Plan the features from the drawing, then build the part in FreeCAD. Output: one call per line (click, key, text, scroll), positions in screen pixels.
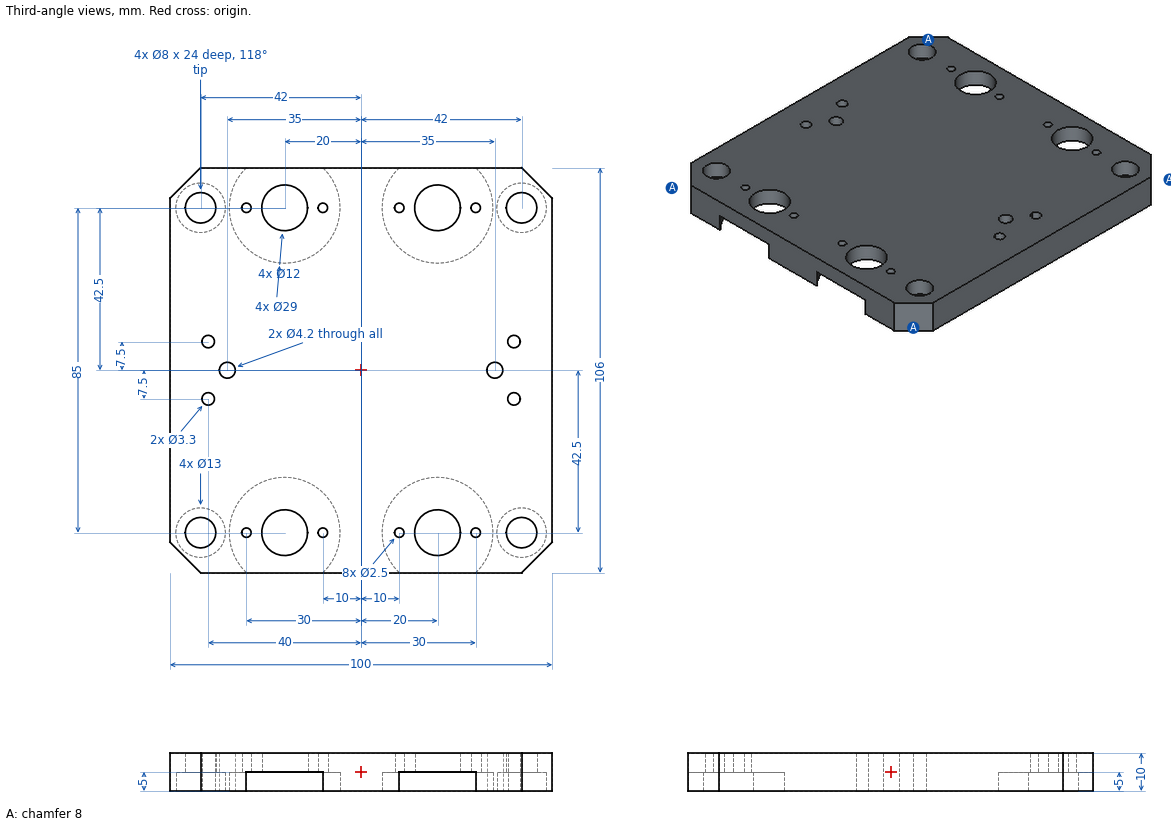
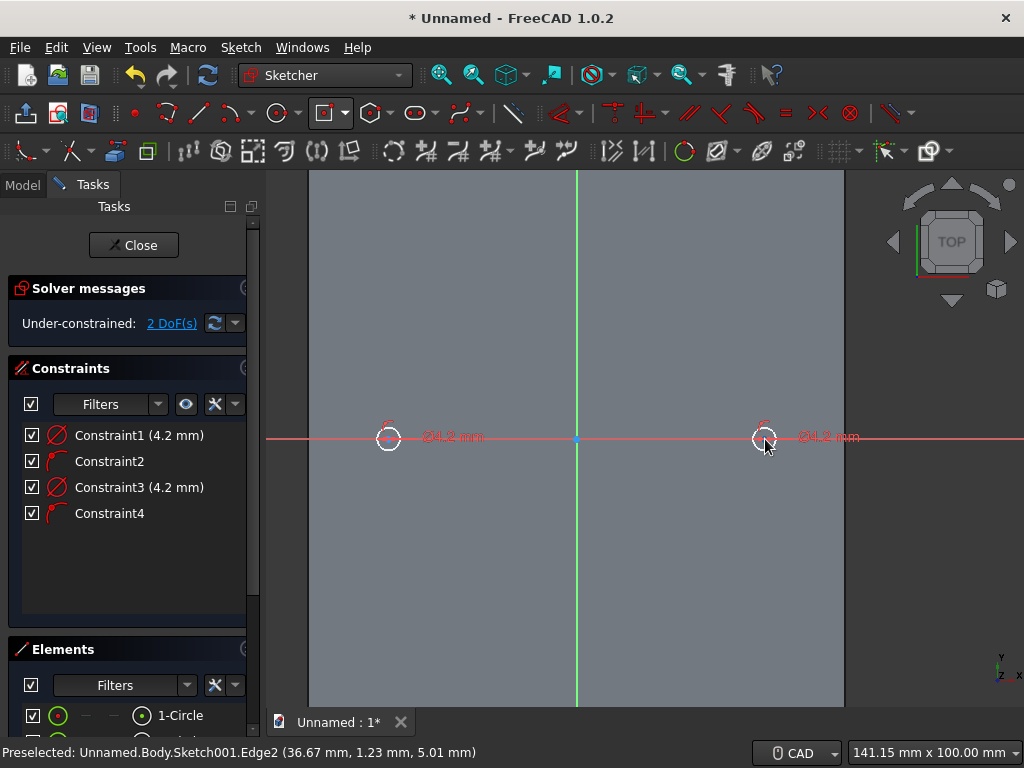
click(389, 439)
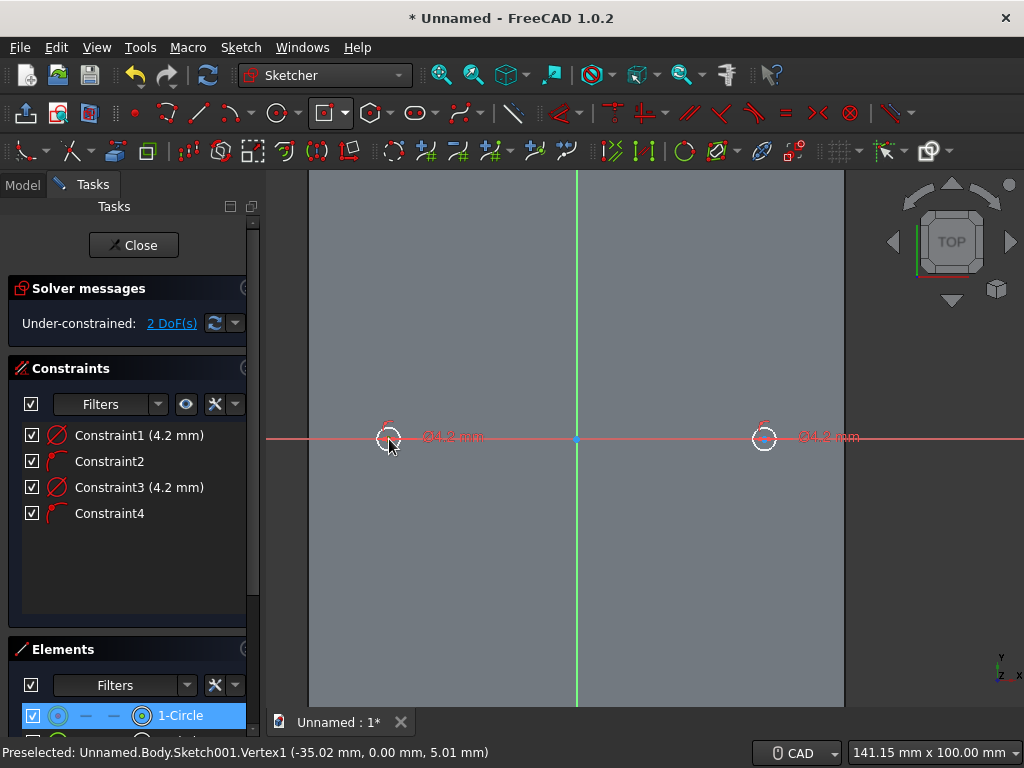
click(582, 114)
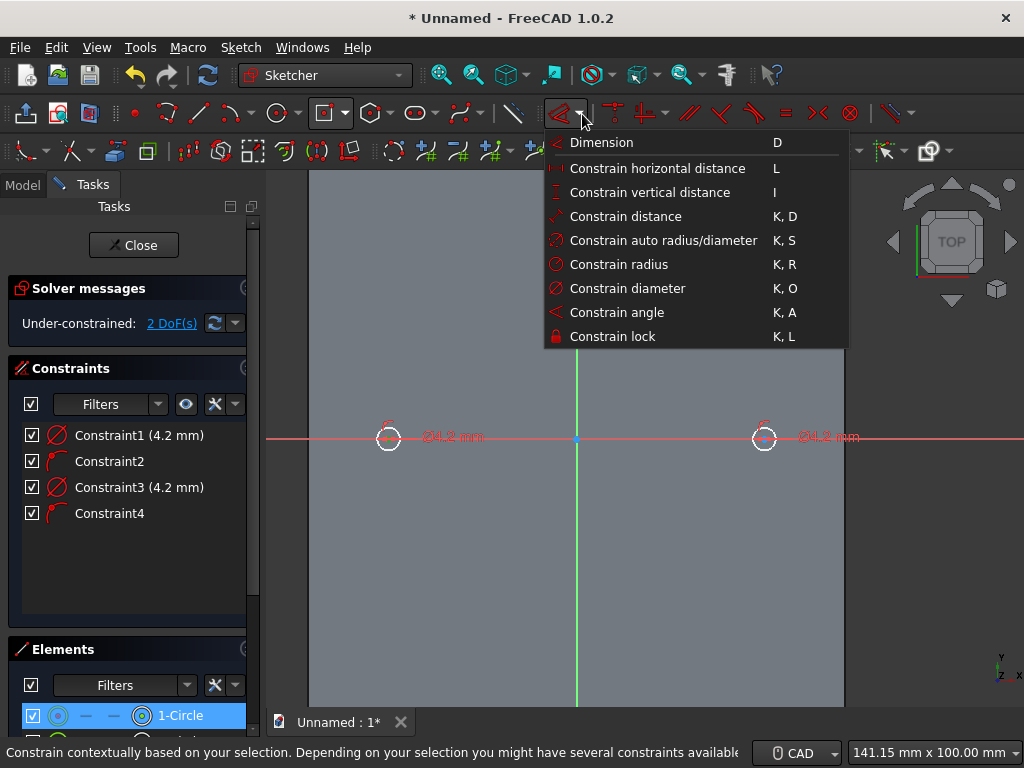
click(697, 168)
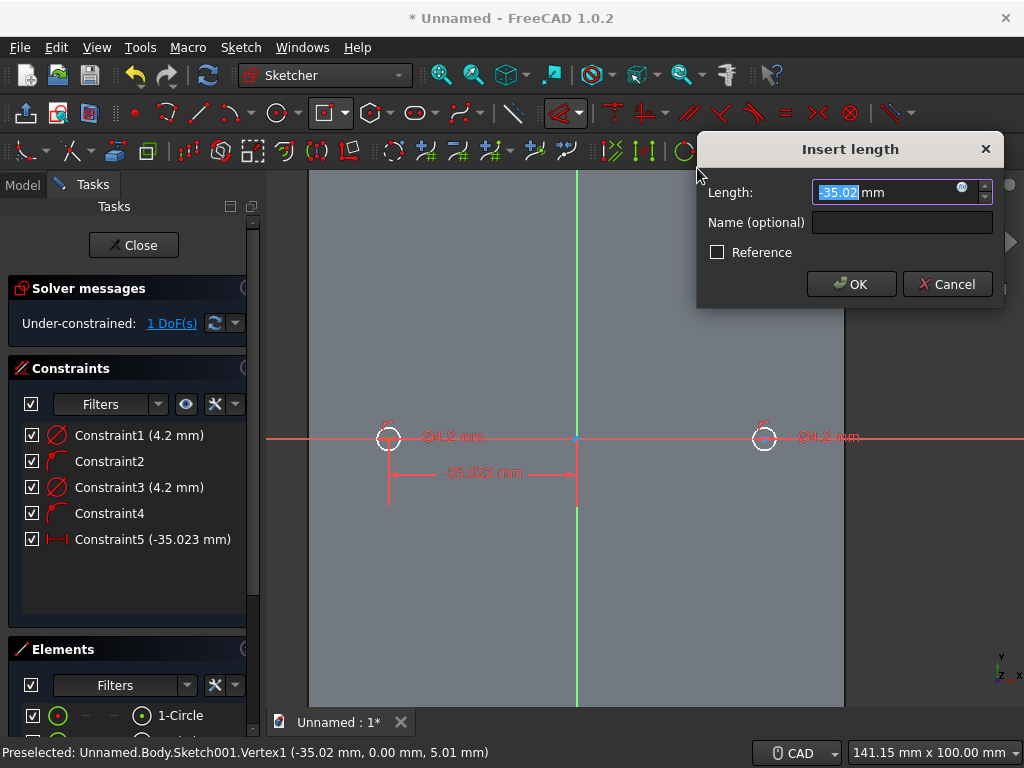
text(-35)
key(Return)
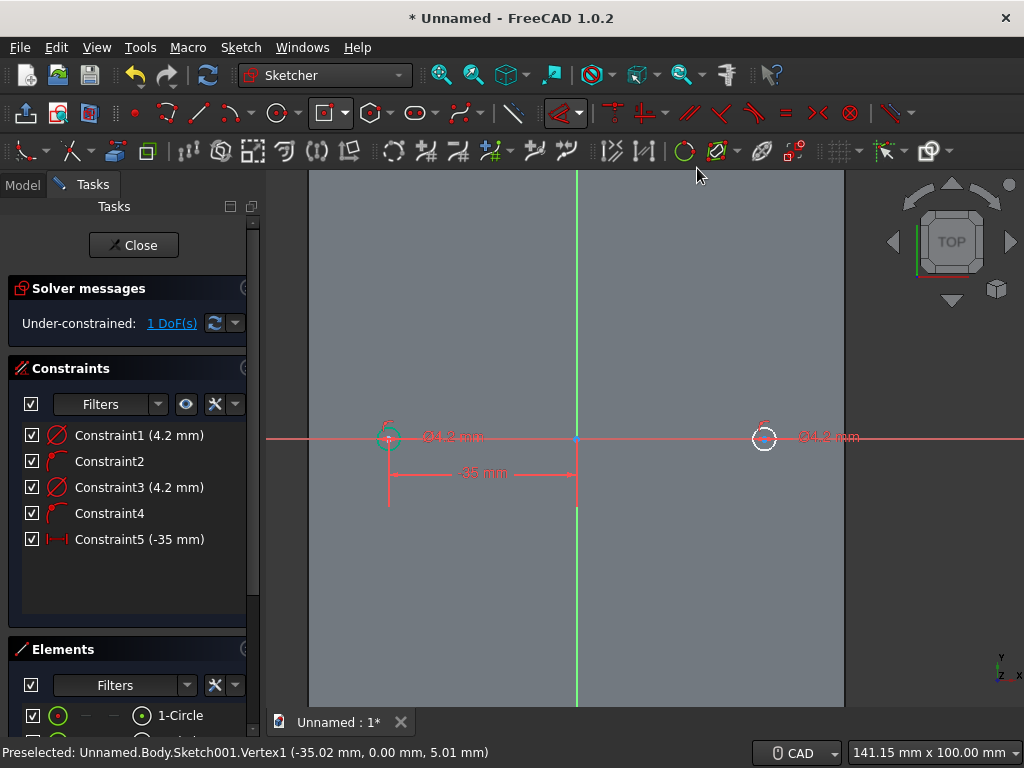
click(764, 439)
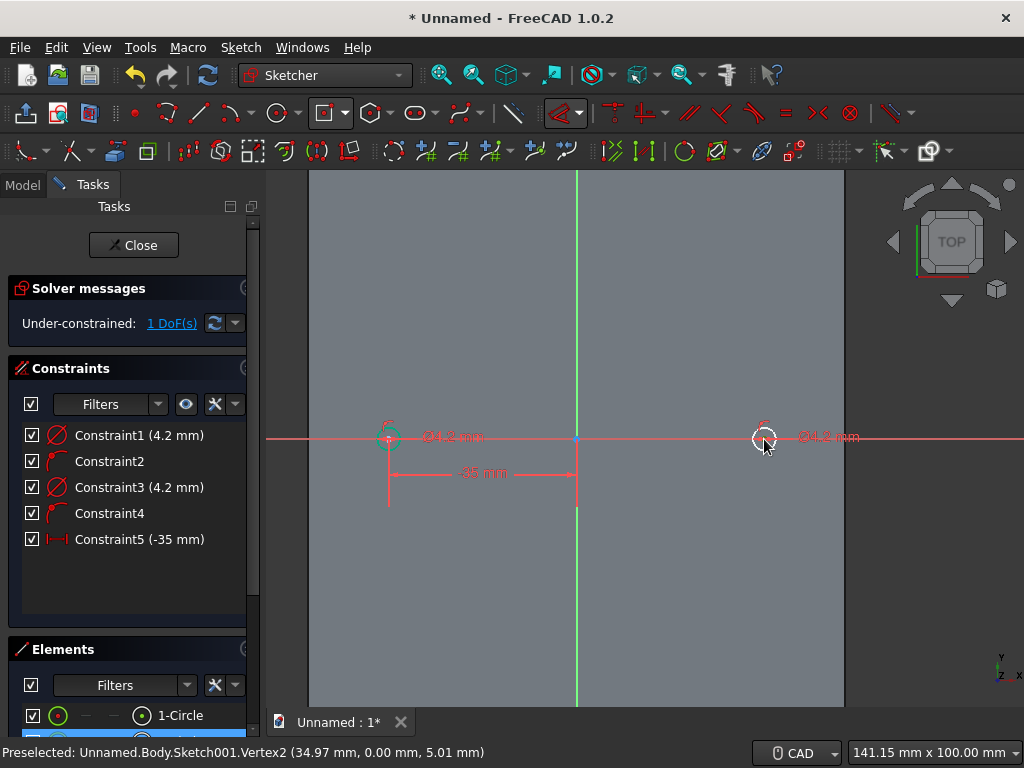
click(582, 114)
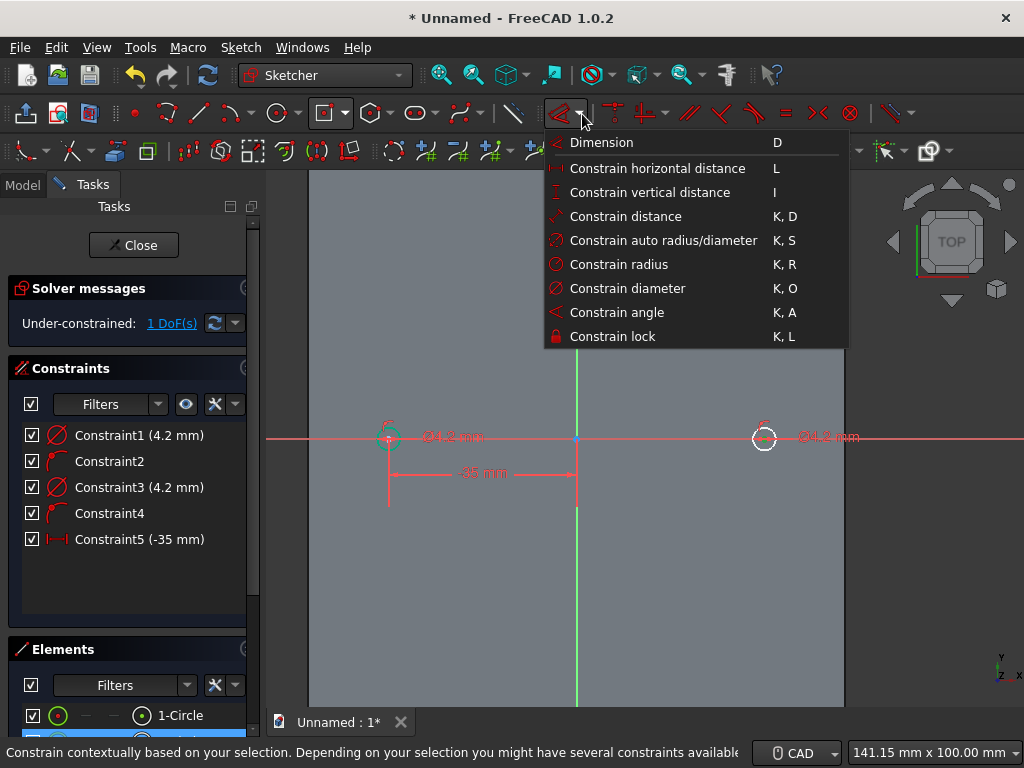
click(697, 168)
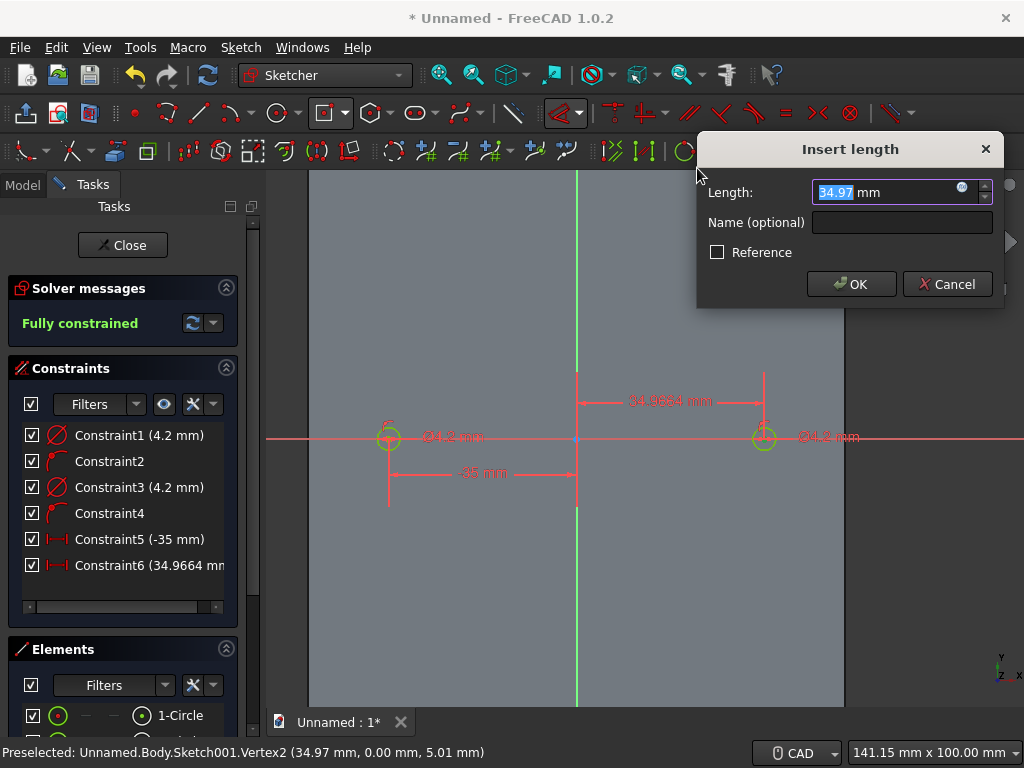
text(35)
key(Return)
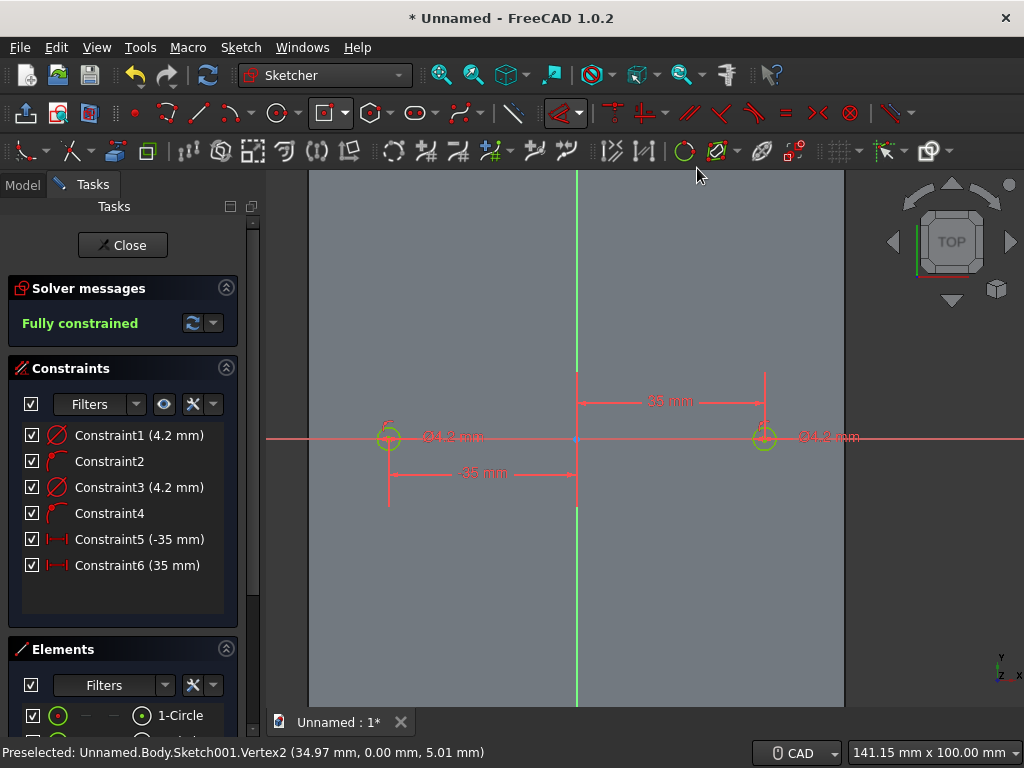
click(123, 245)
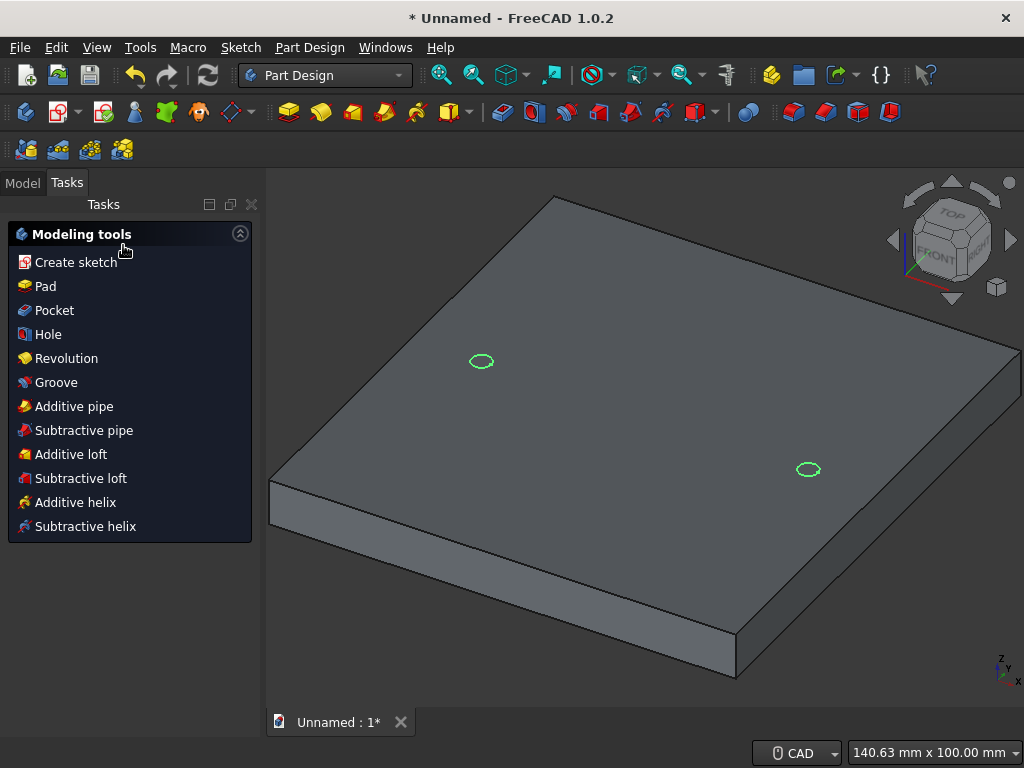
click(536, 112)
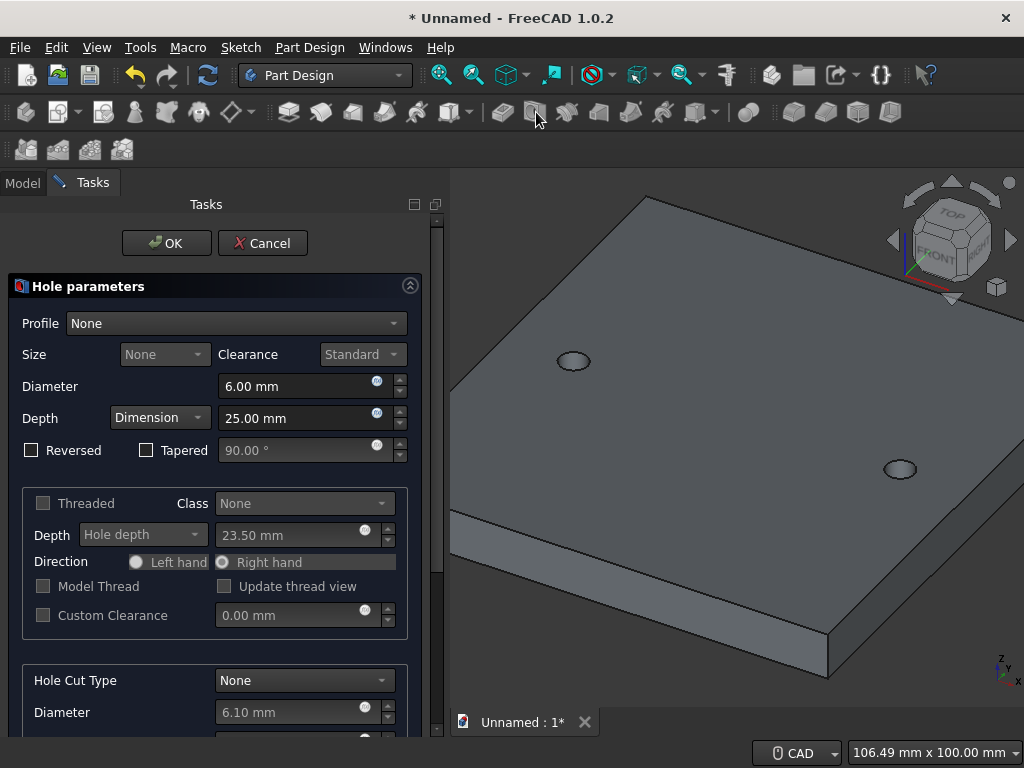
triple_click(305, 386)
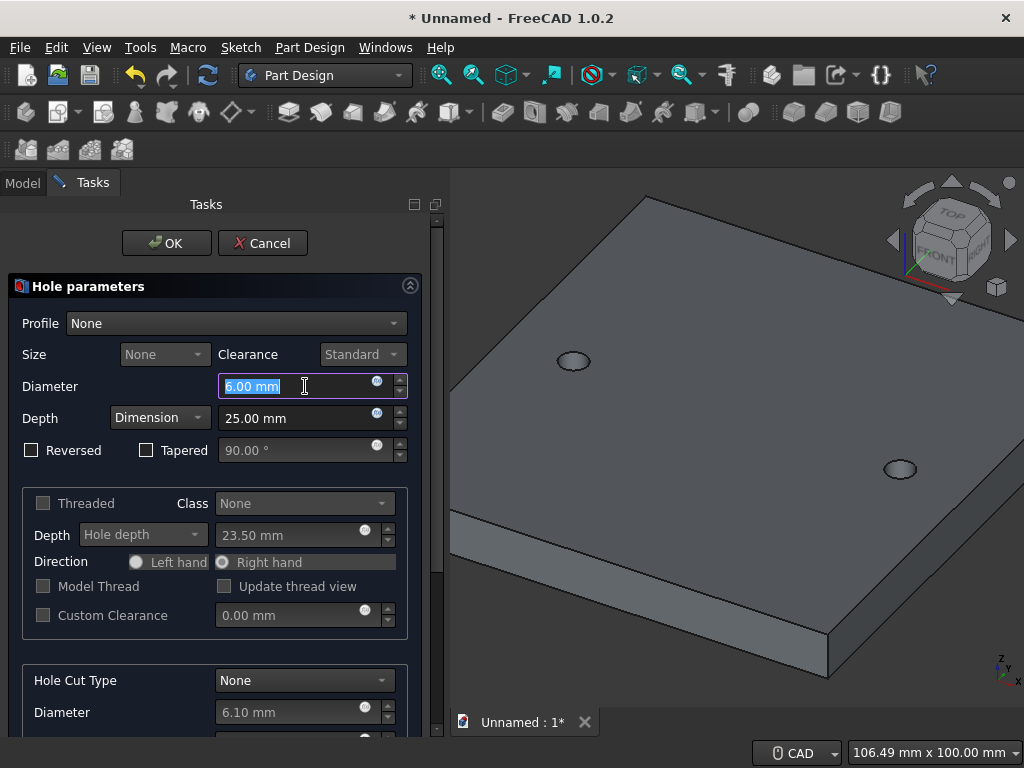
text(4.2)
key(Tab)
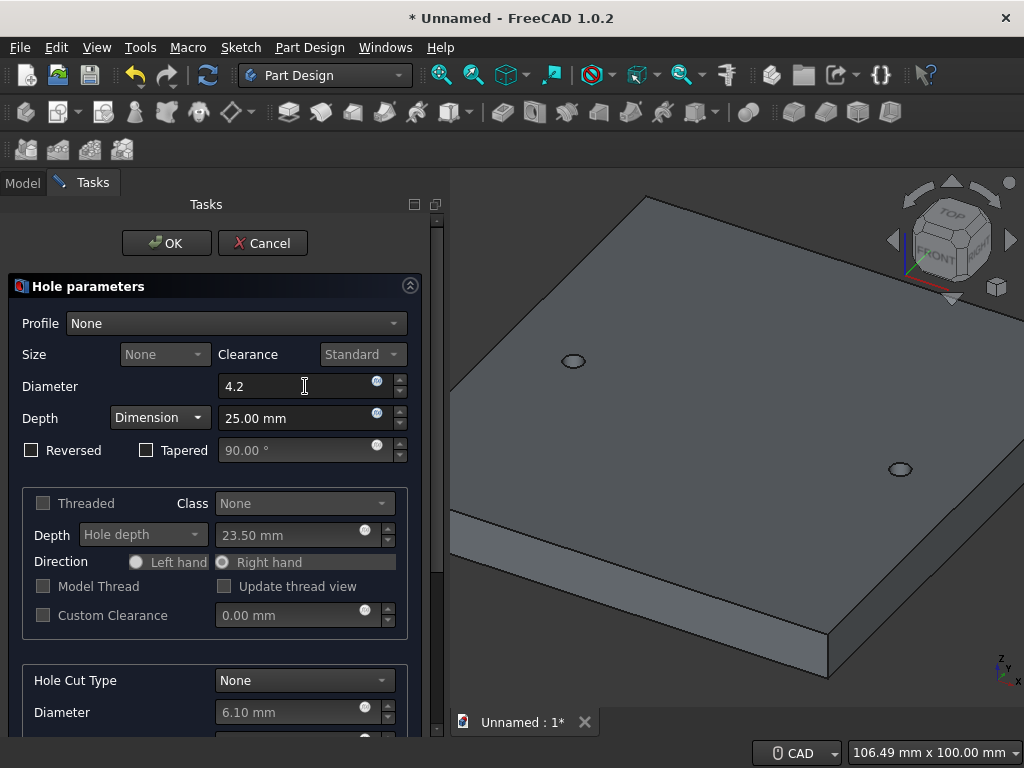
click(161, 418)